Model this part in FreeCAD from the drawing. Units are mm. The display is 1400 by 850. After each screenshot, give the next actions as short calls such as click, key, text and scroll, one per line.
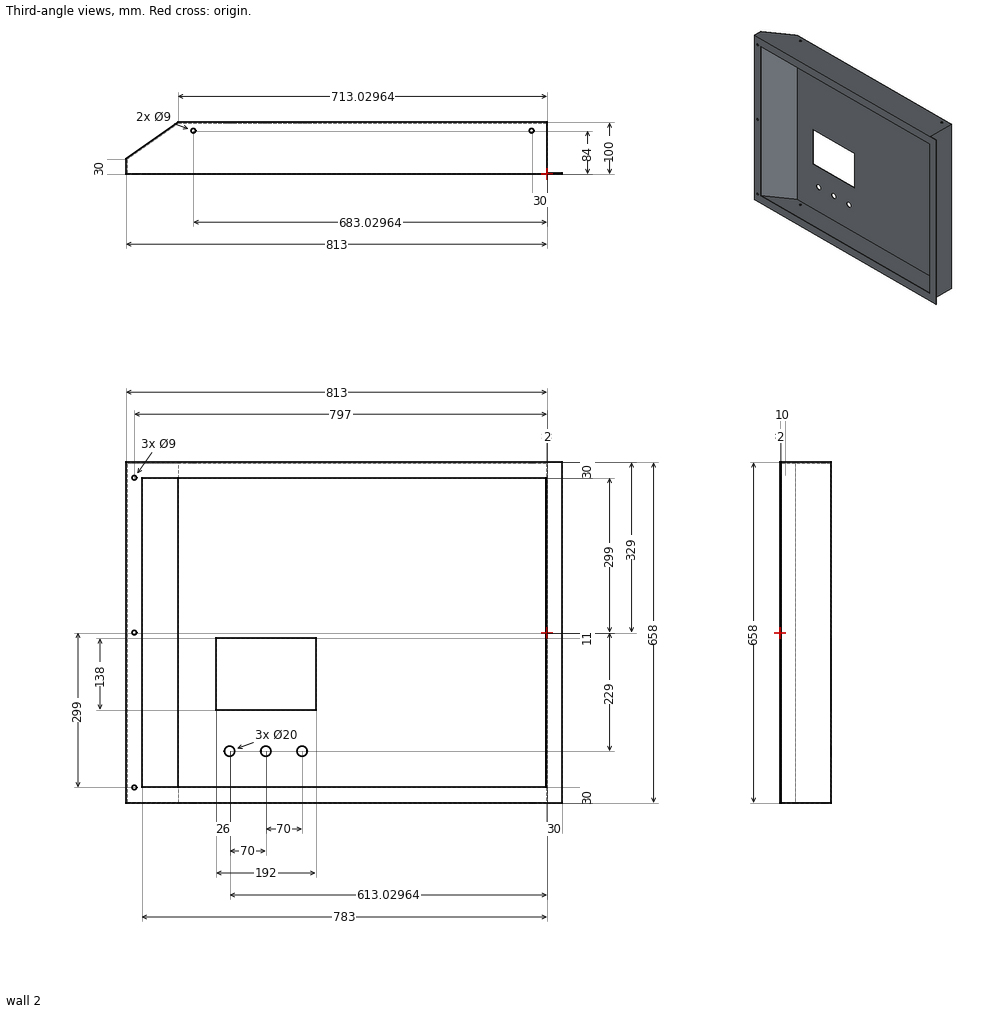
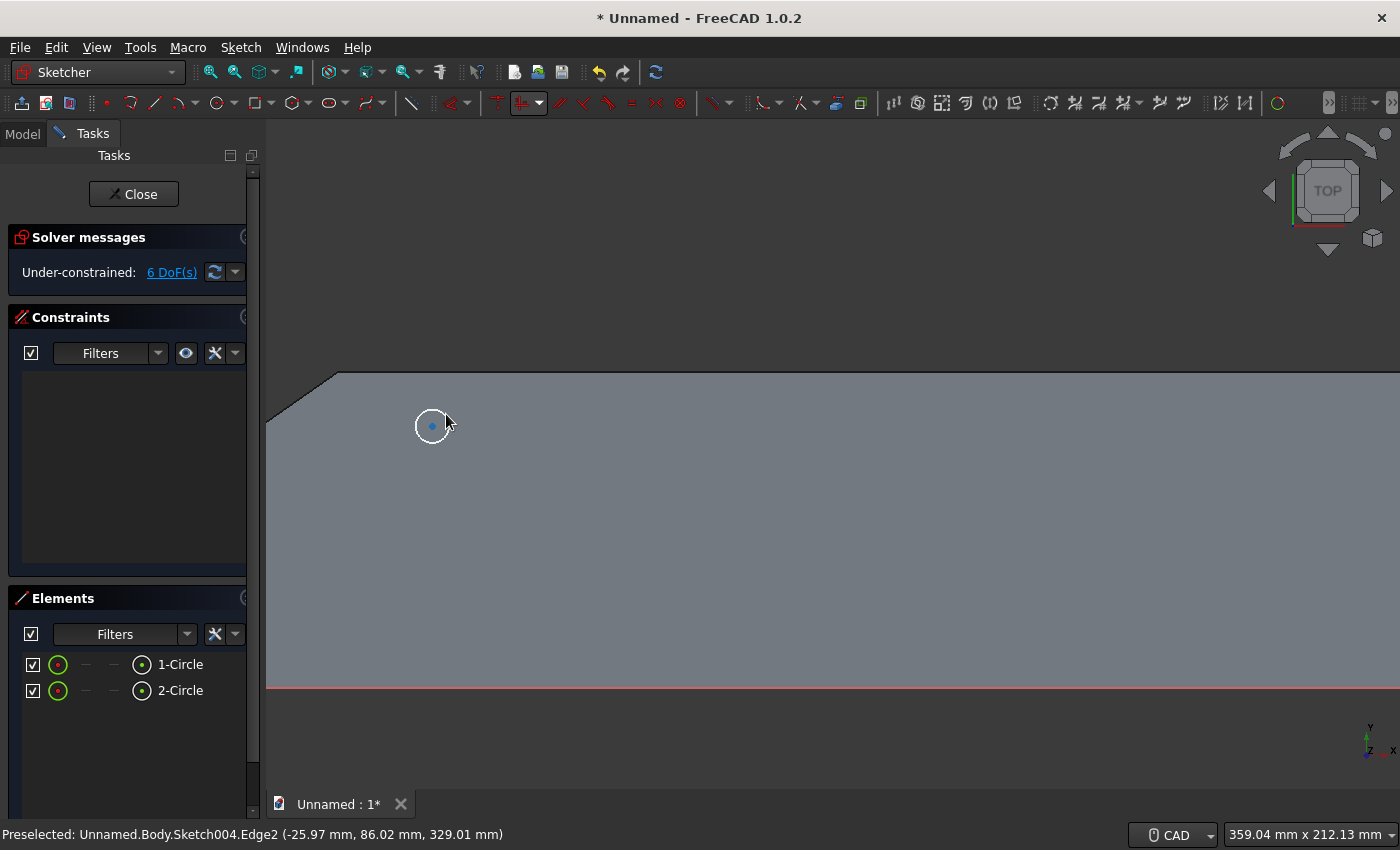
click(444, 414)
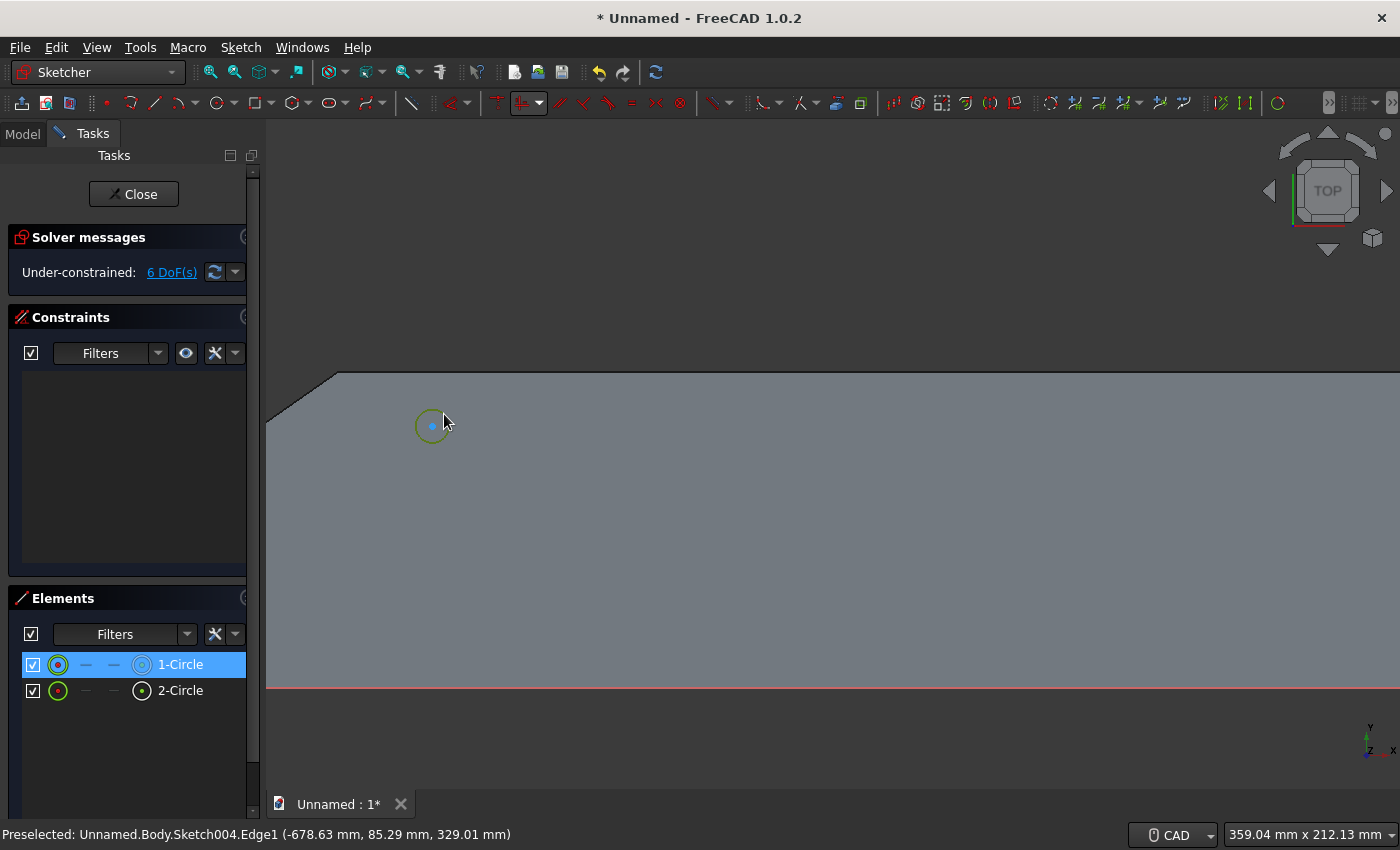
scroll(446, 414, down, 6)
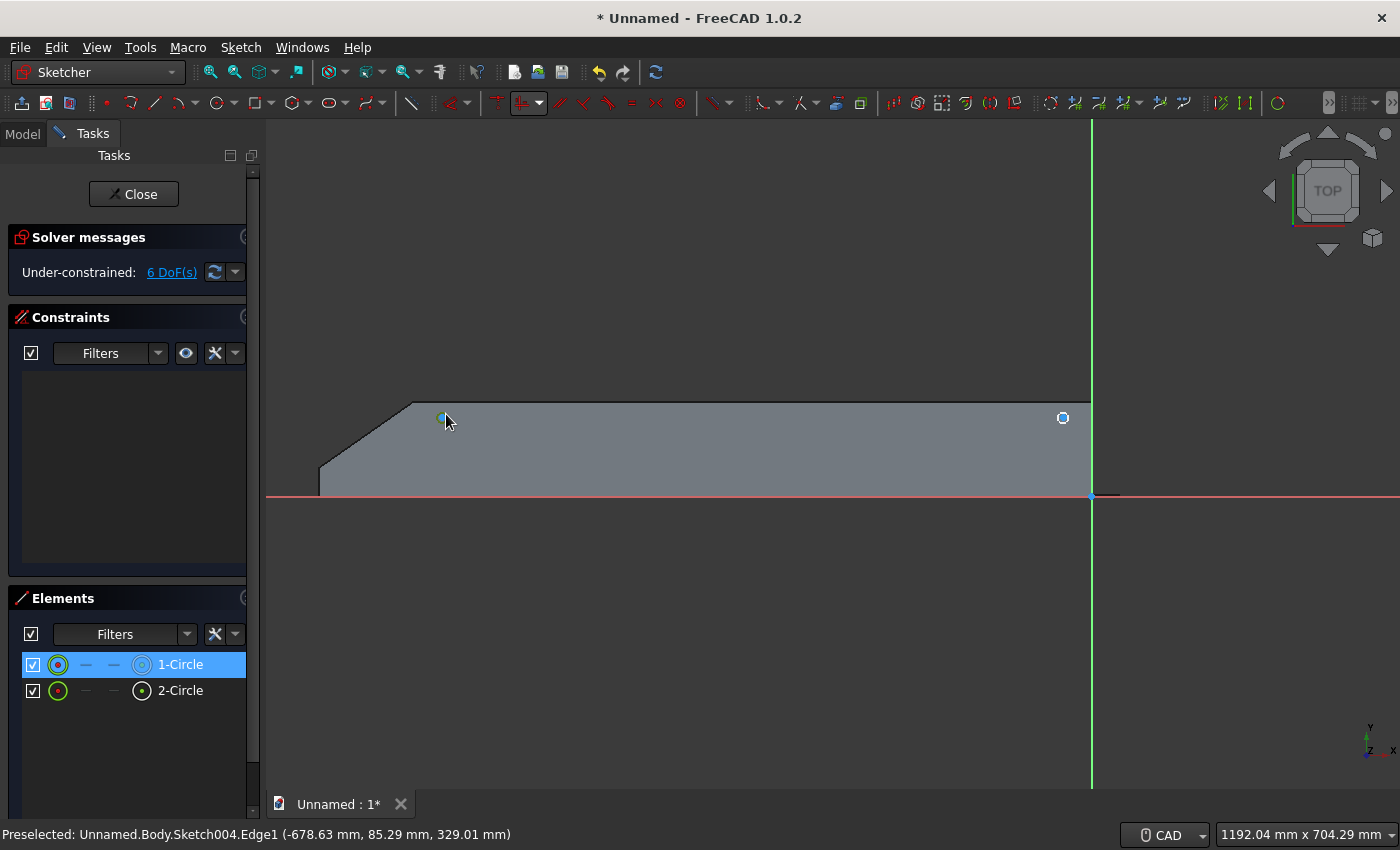
scroll(1067, 414, up, 5)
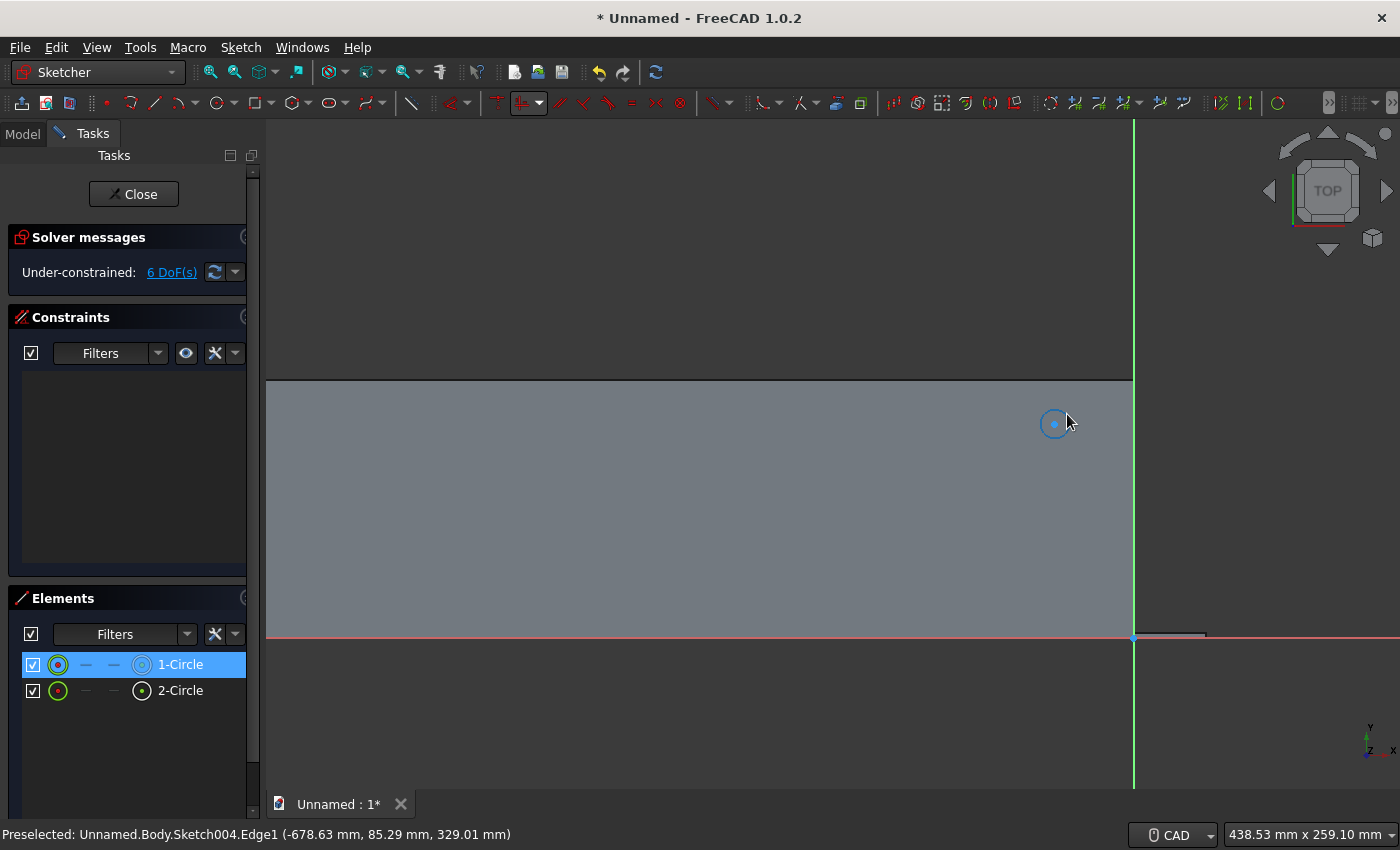
click(1065, 414)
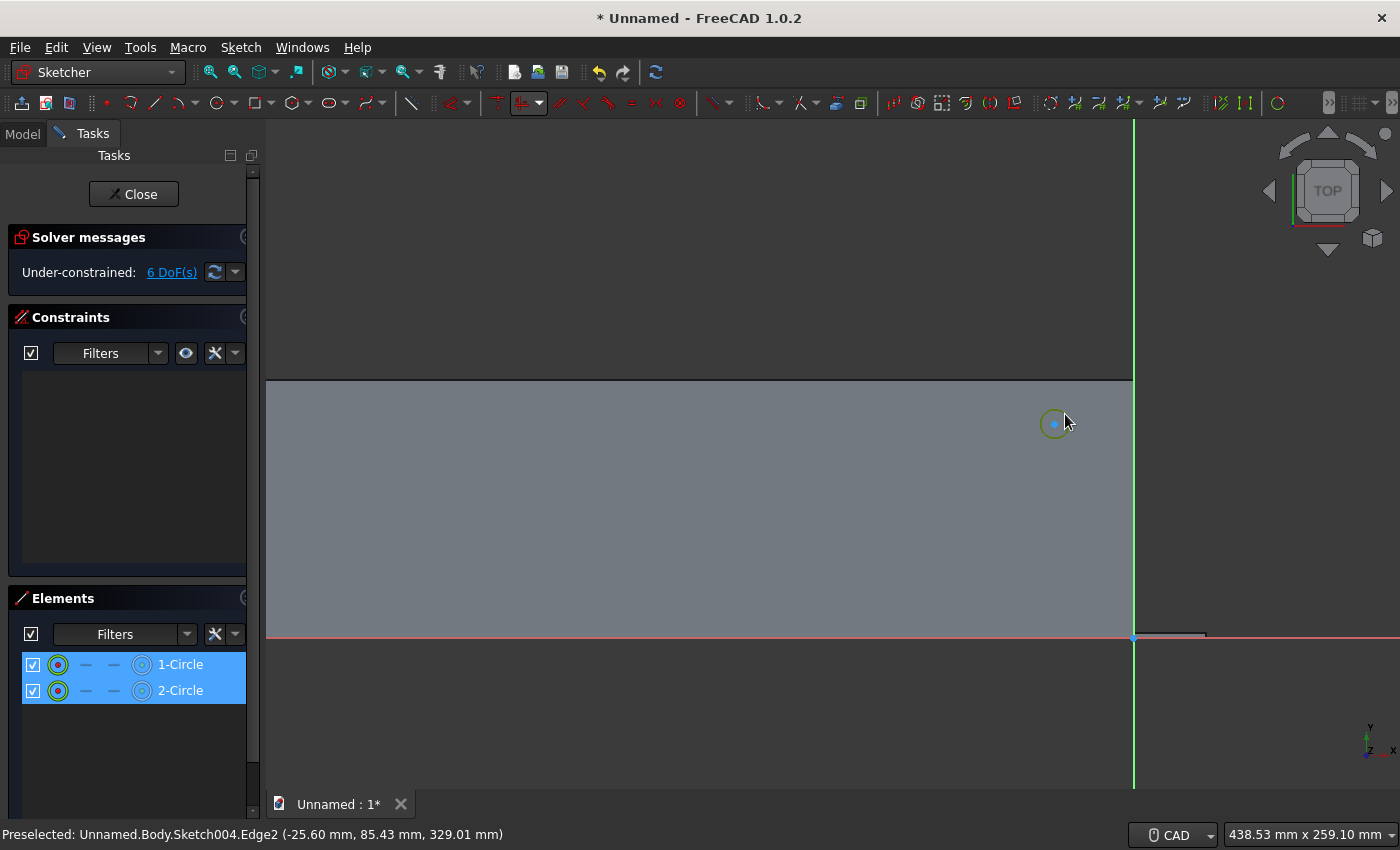
click(632, 104)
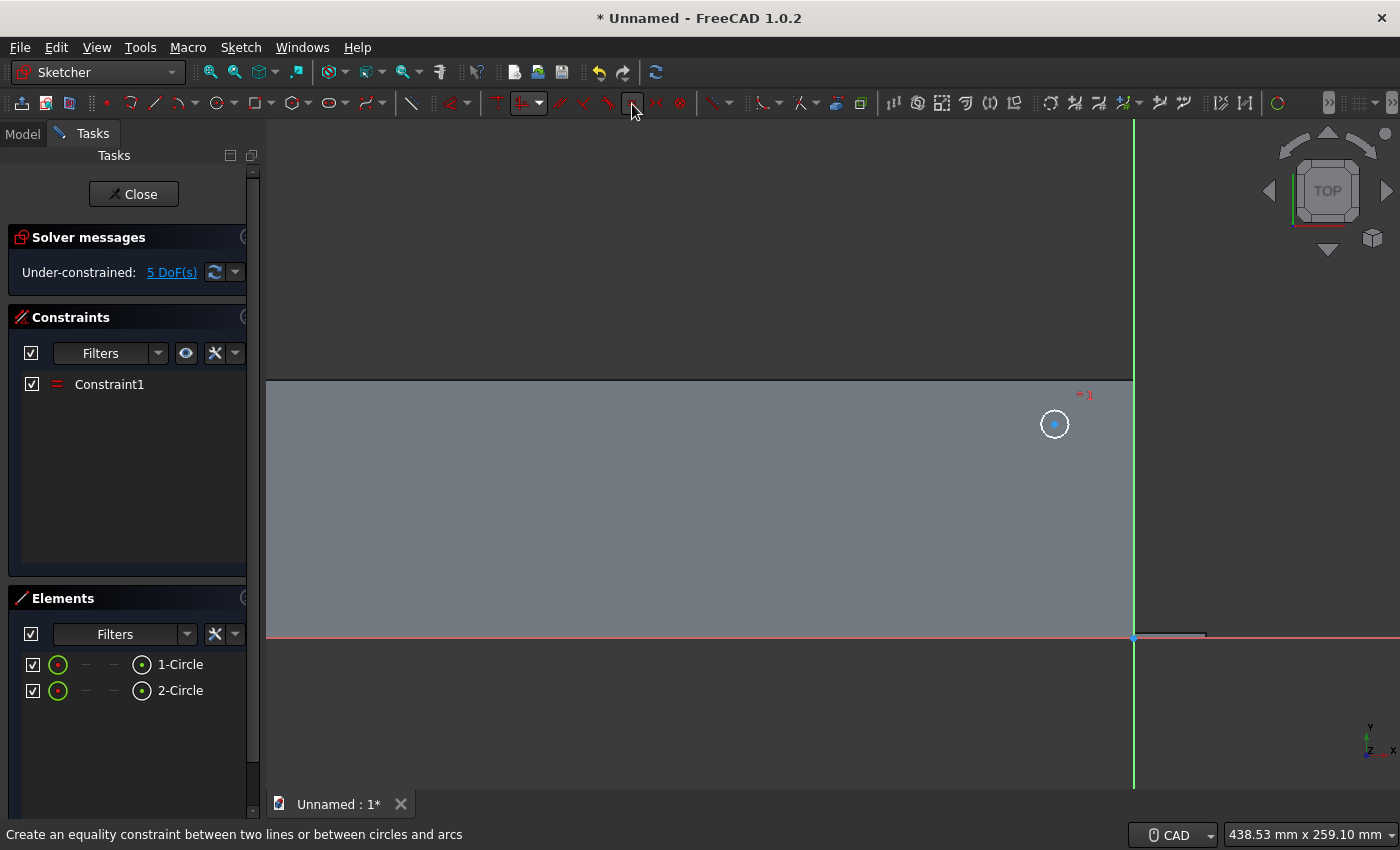
scroll(1067, 413, down, 5)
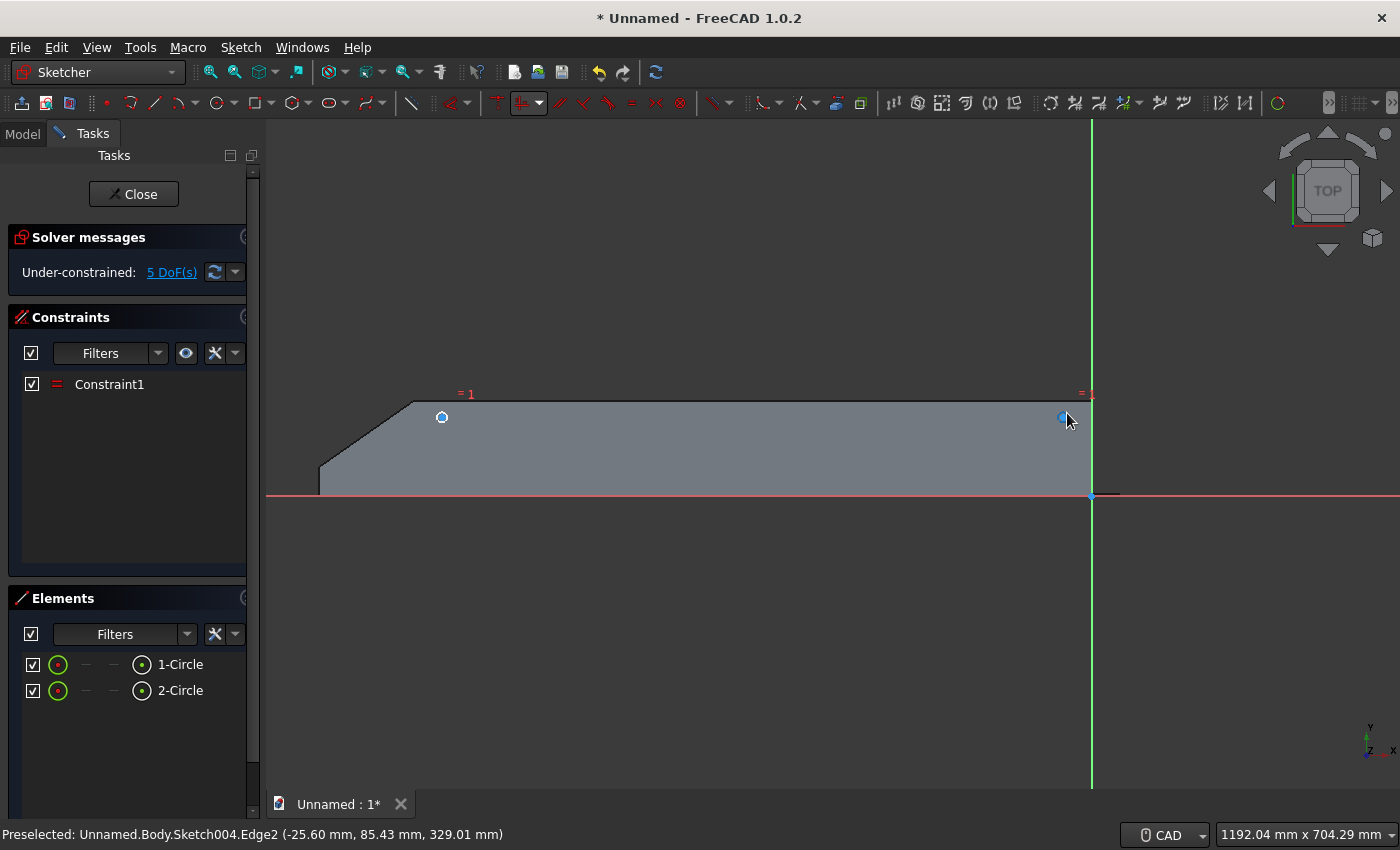
click(442, 417)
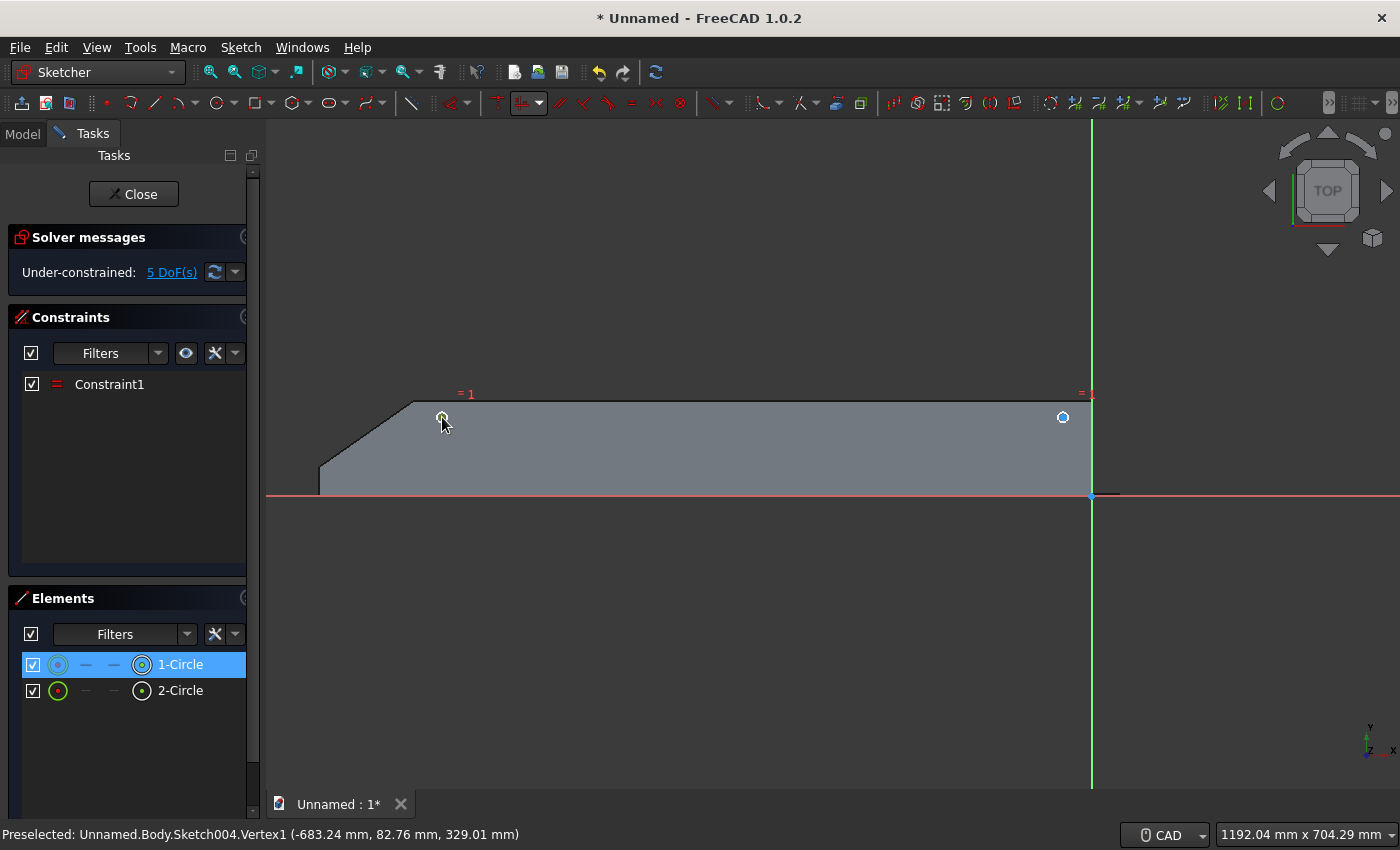
click(1063, 417)